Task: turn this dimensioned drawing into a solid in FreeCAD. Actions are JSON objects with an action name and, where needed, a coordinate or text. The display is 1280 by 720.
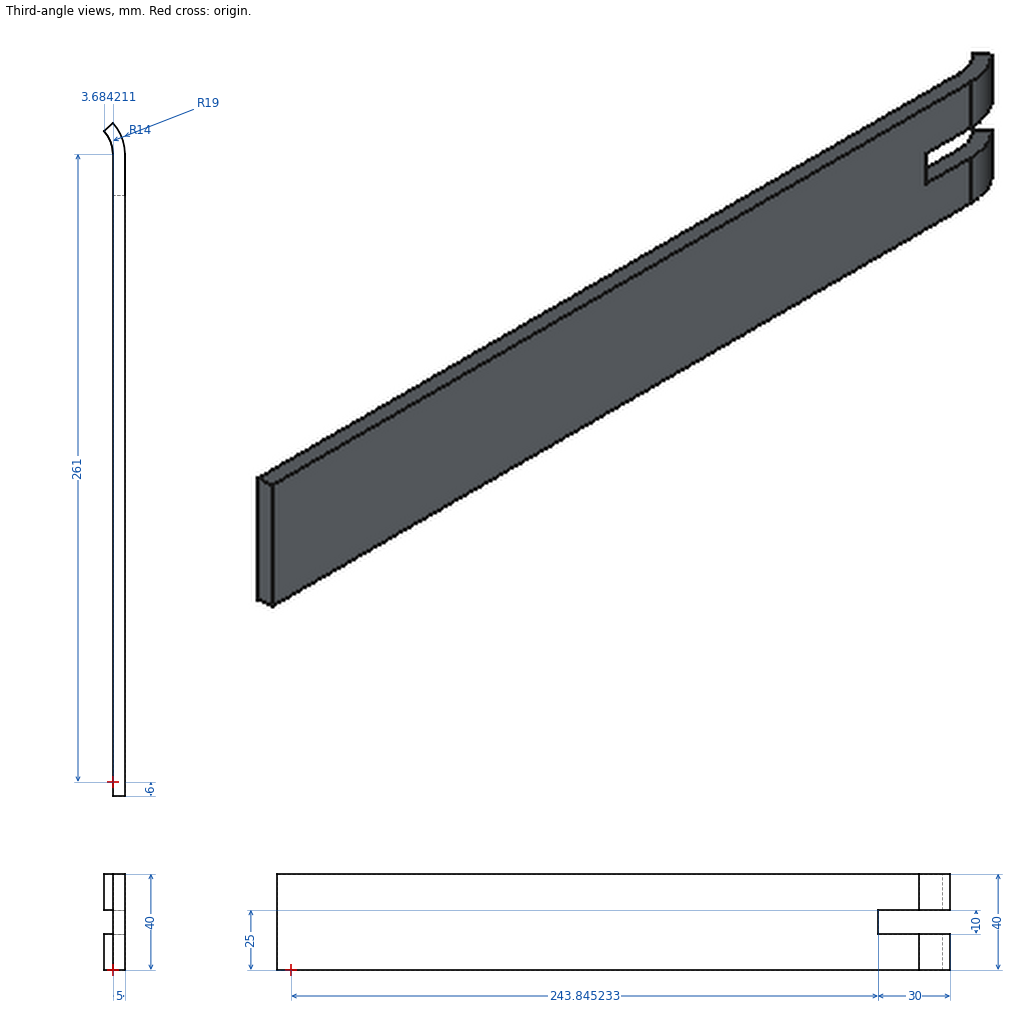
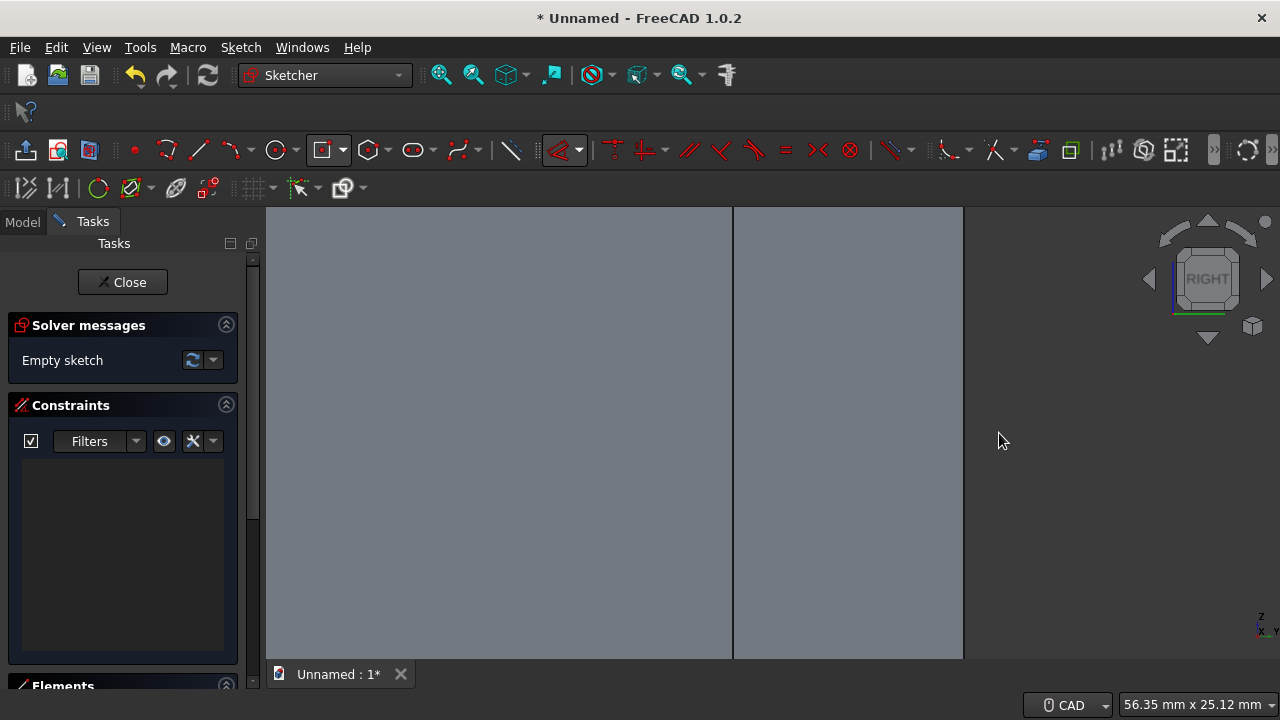
{"action": "key", "text": "g r"}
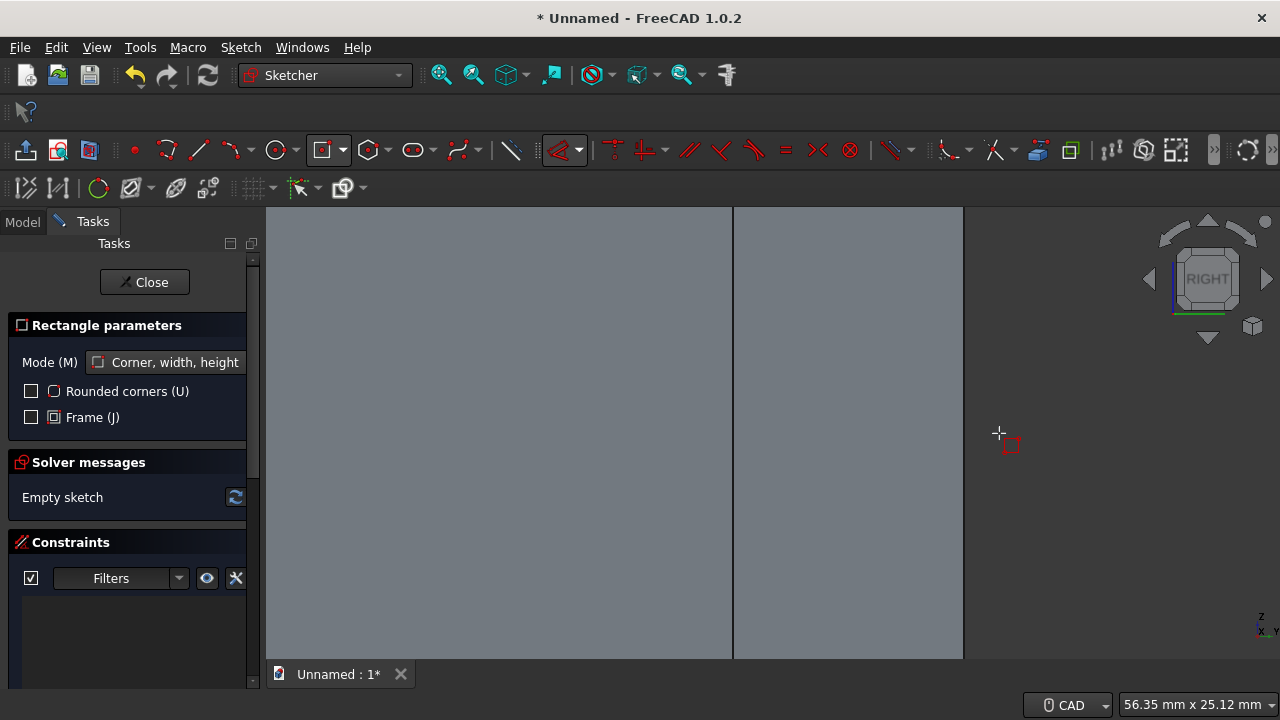
{"action": "left_click", "coordinate": [425, 338]}
{"action": "mouse_move", "coordinate": [964, 518]}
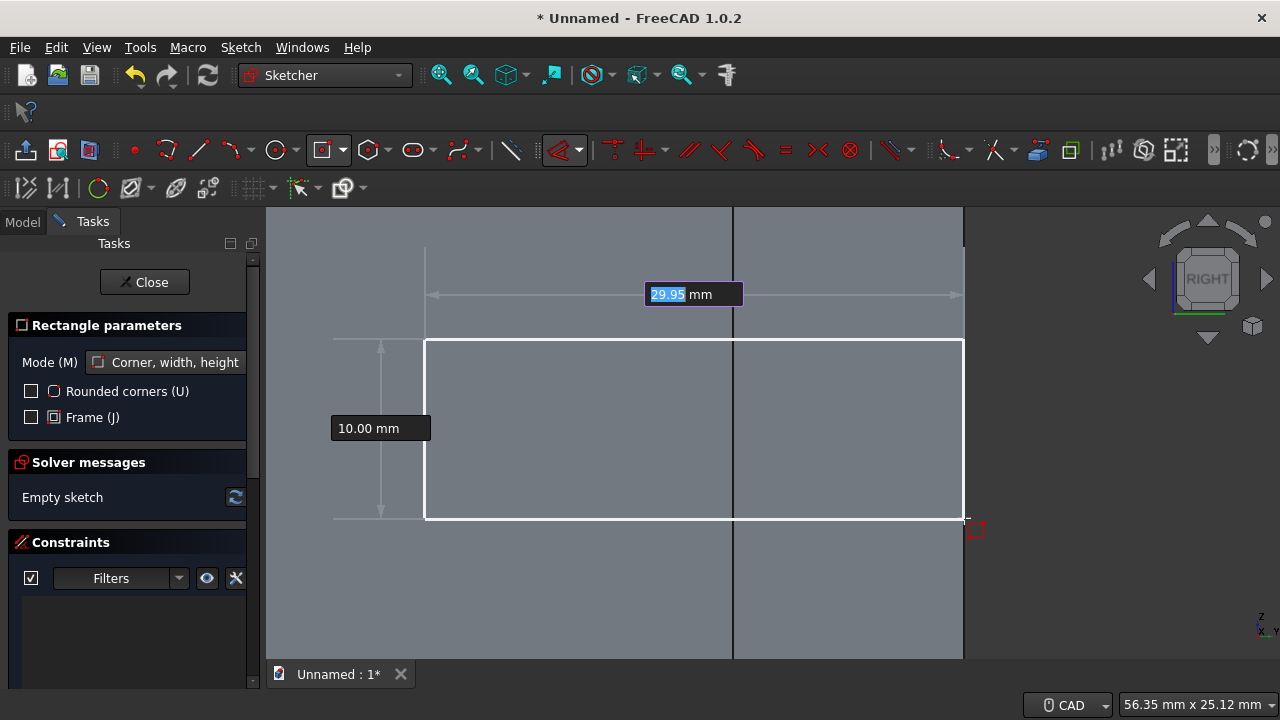
{"action": "type", "text": "30"}
{"action": "key", "text": "Tab"}
{"action": "type", "text": "10"}
{"action": "key", "text": "Return"}
{"action": "key", "text": "Escape"}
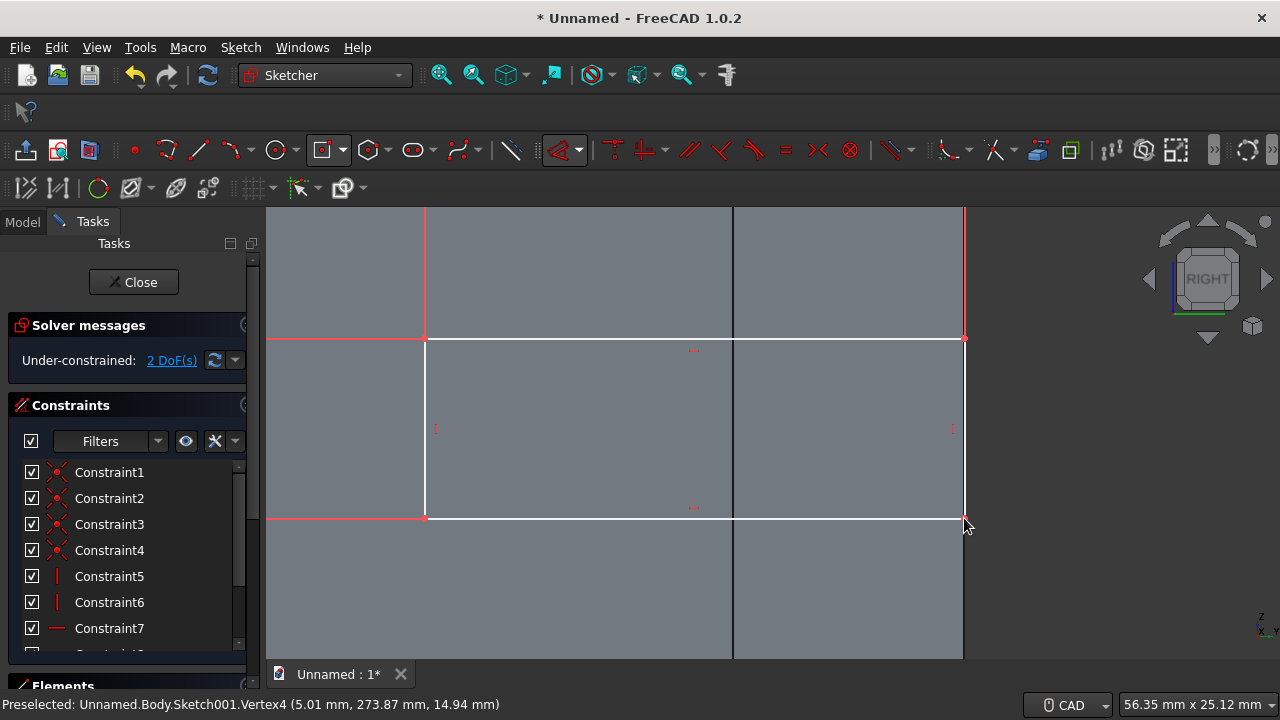
{"action": "left_click", "coordinate": [425, 339]}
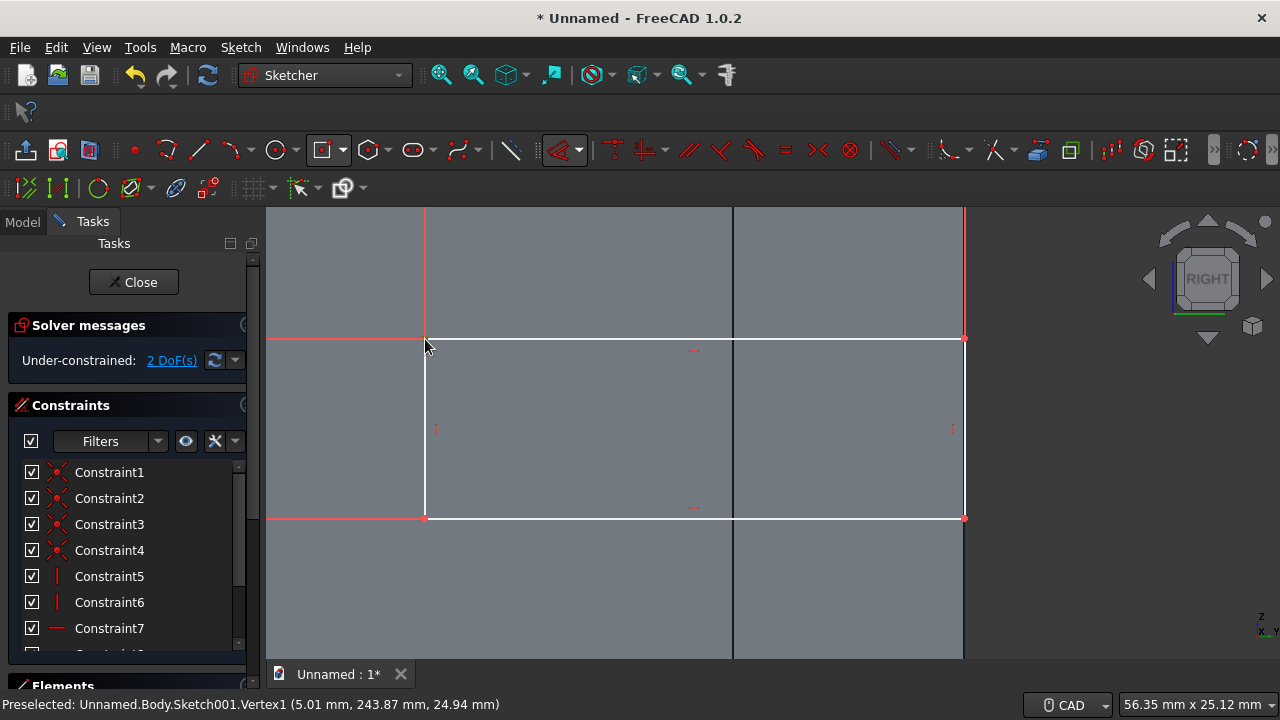
{"action": "left_click", "coordinate": [582, 150]}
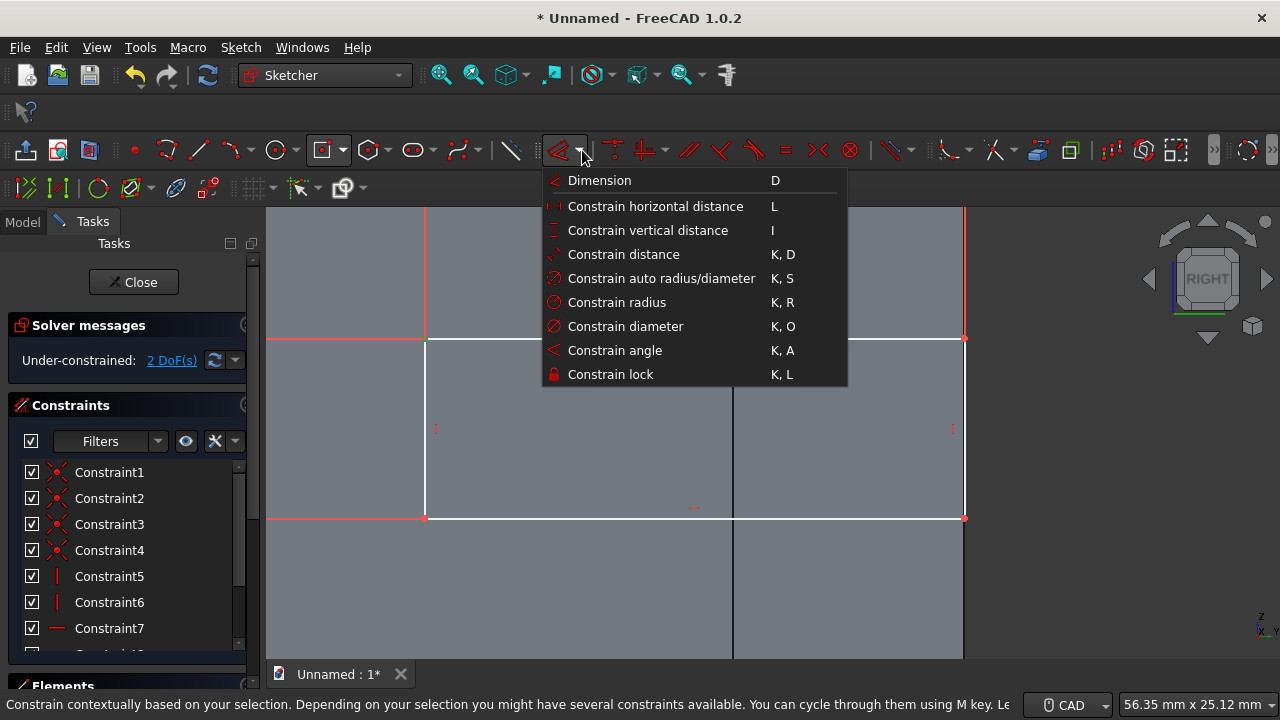
{"action": "left_click", "coordinate": [695, 230]}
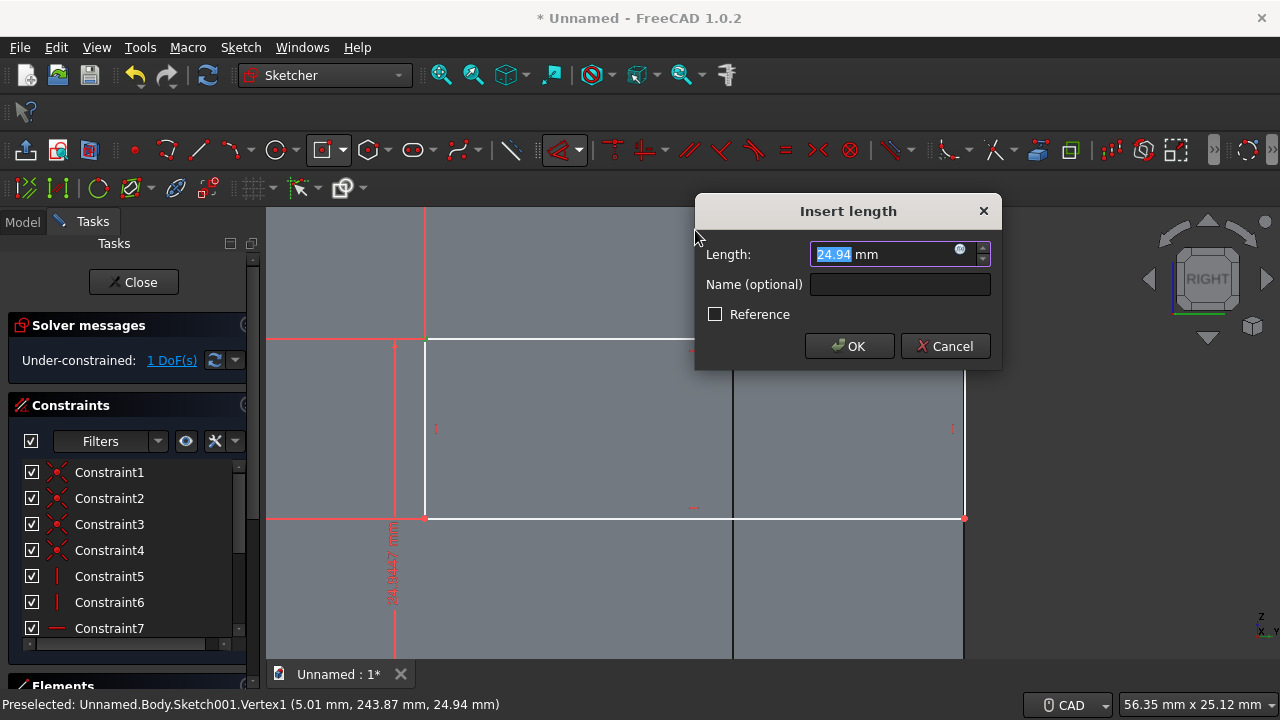
{"action": "type", "text": "25"}
{"action": "key", "text": "Return"}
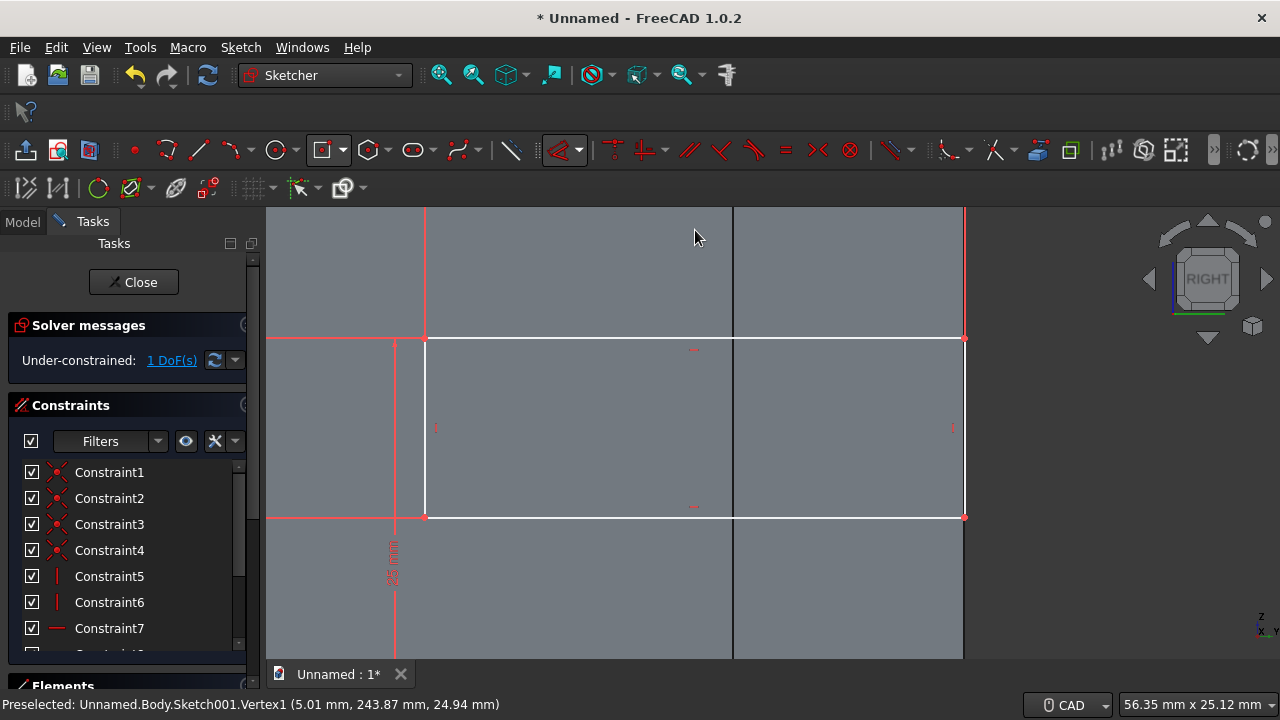
{"action": "left_click", "coordinate": [425, 338]}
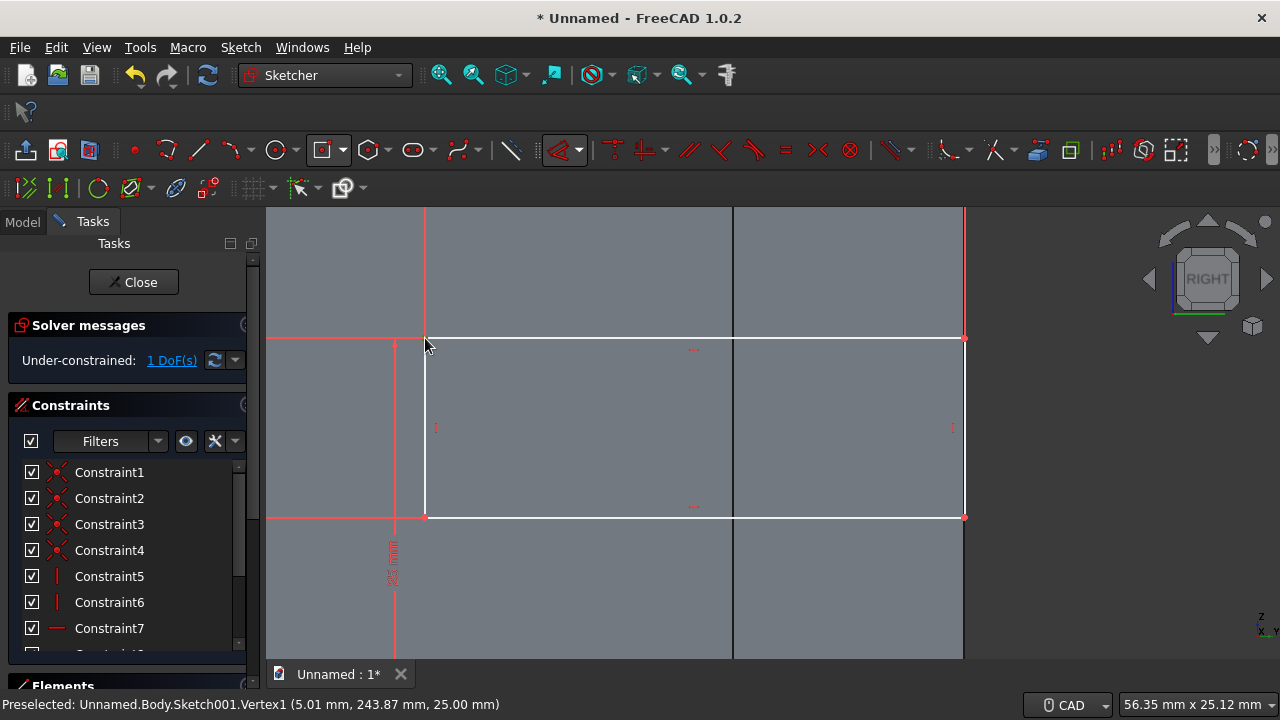
{"action": "key", "text": "l"}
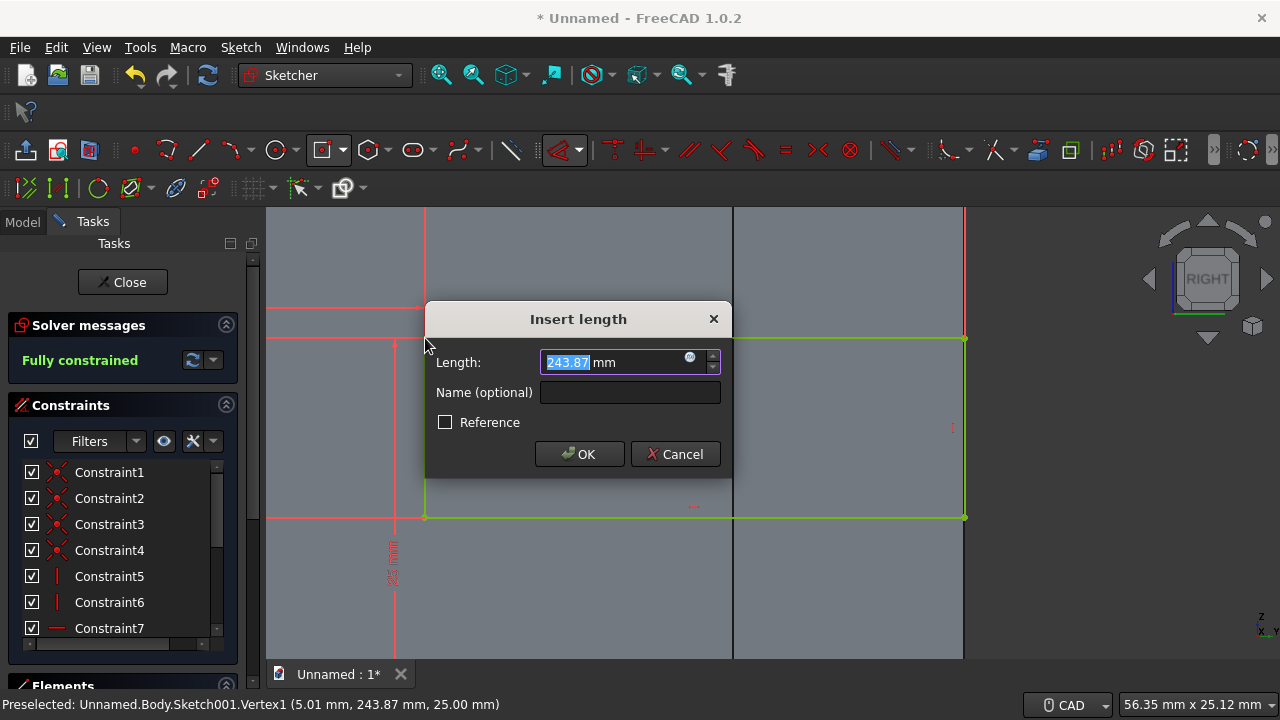
{"action": "type", "text": "243.845233"}
{"action": "key", "text": "Return"}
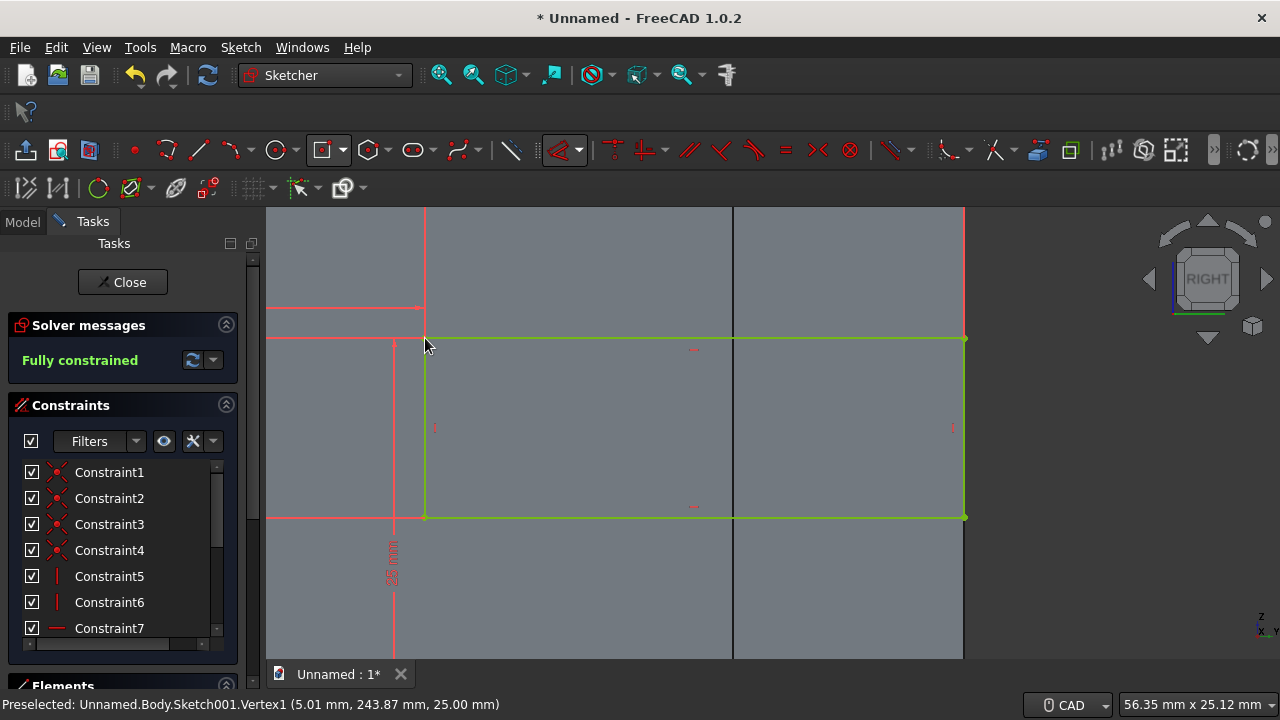
{"action": "left_click", "coordinate": [123, 282]}